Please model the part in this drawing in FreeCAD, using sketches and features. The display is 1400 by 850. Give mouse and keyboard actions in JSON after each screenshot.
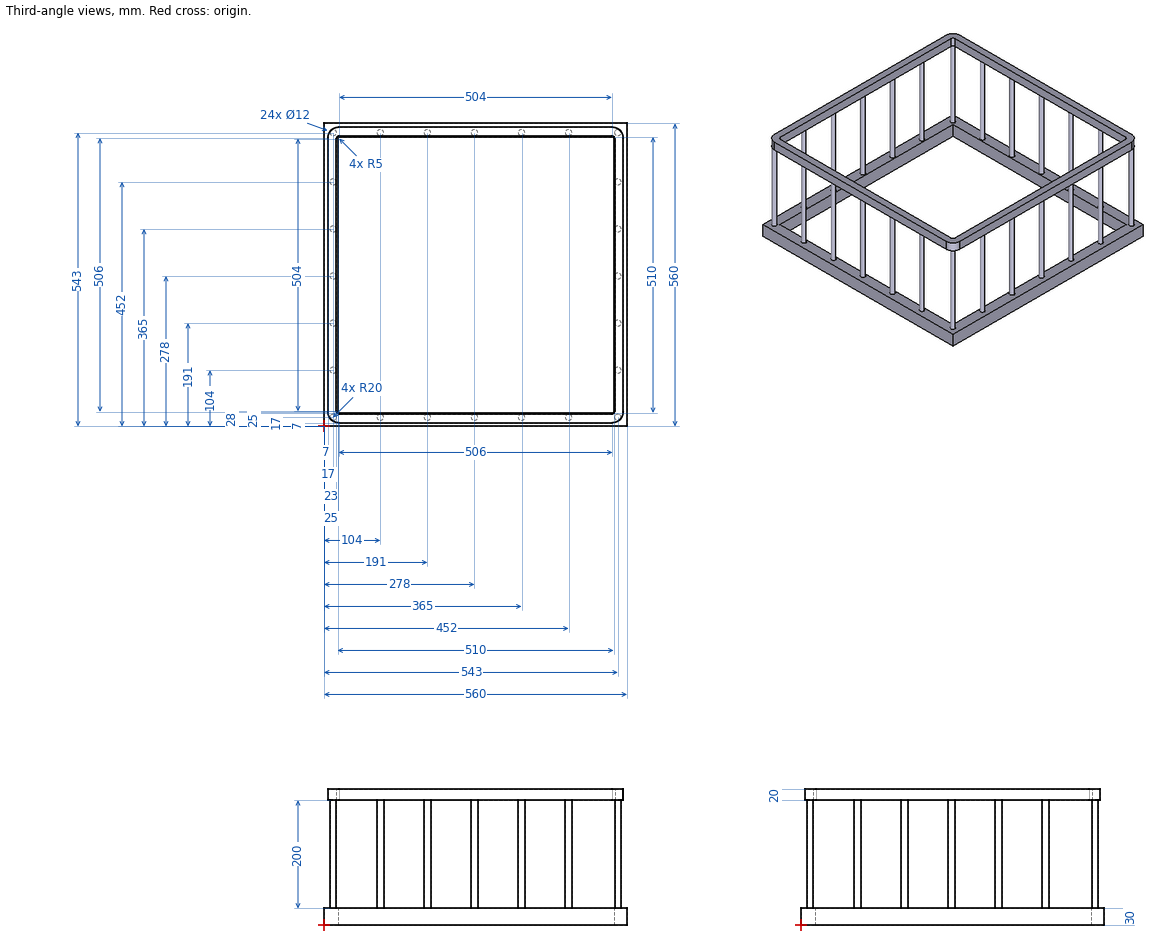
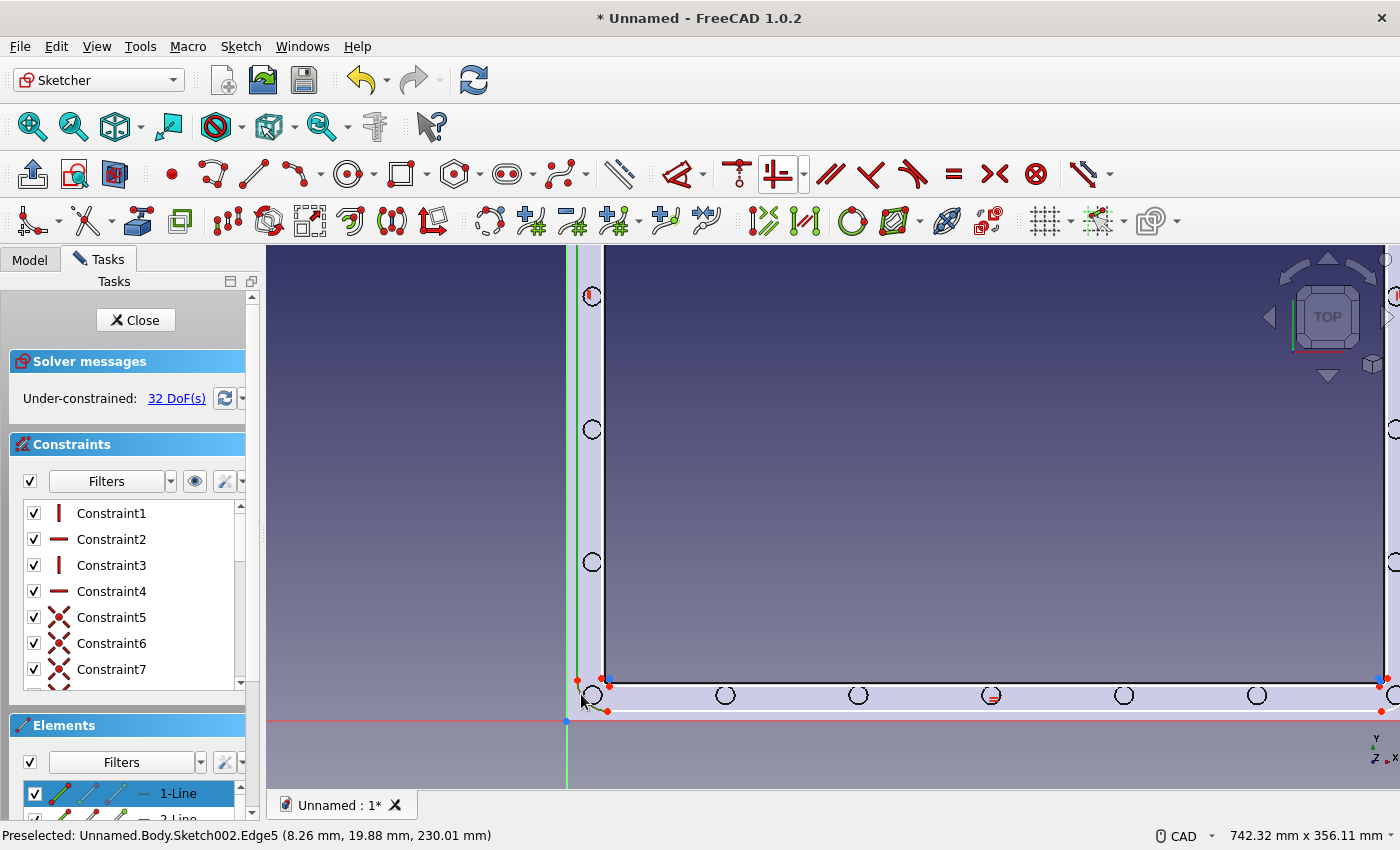
{"action": "left_click", "coordinate": [913, 174]}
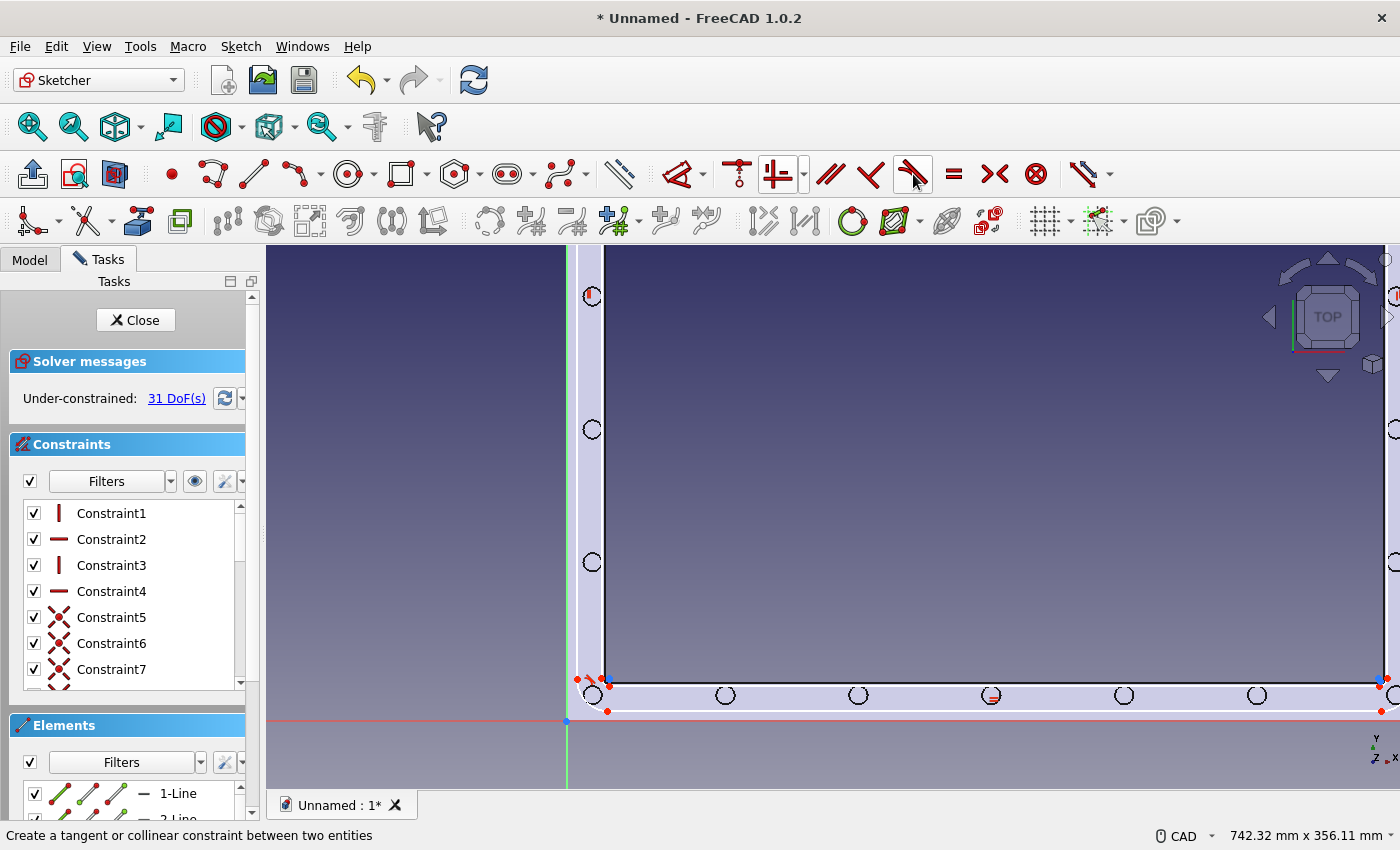
{"action": "scroll", "coordinate": [577, 448], "scroll_direction": "up", "scroll_amount": 2}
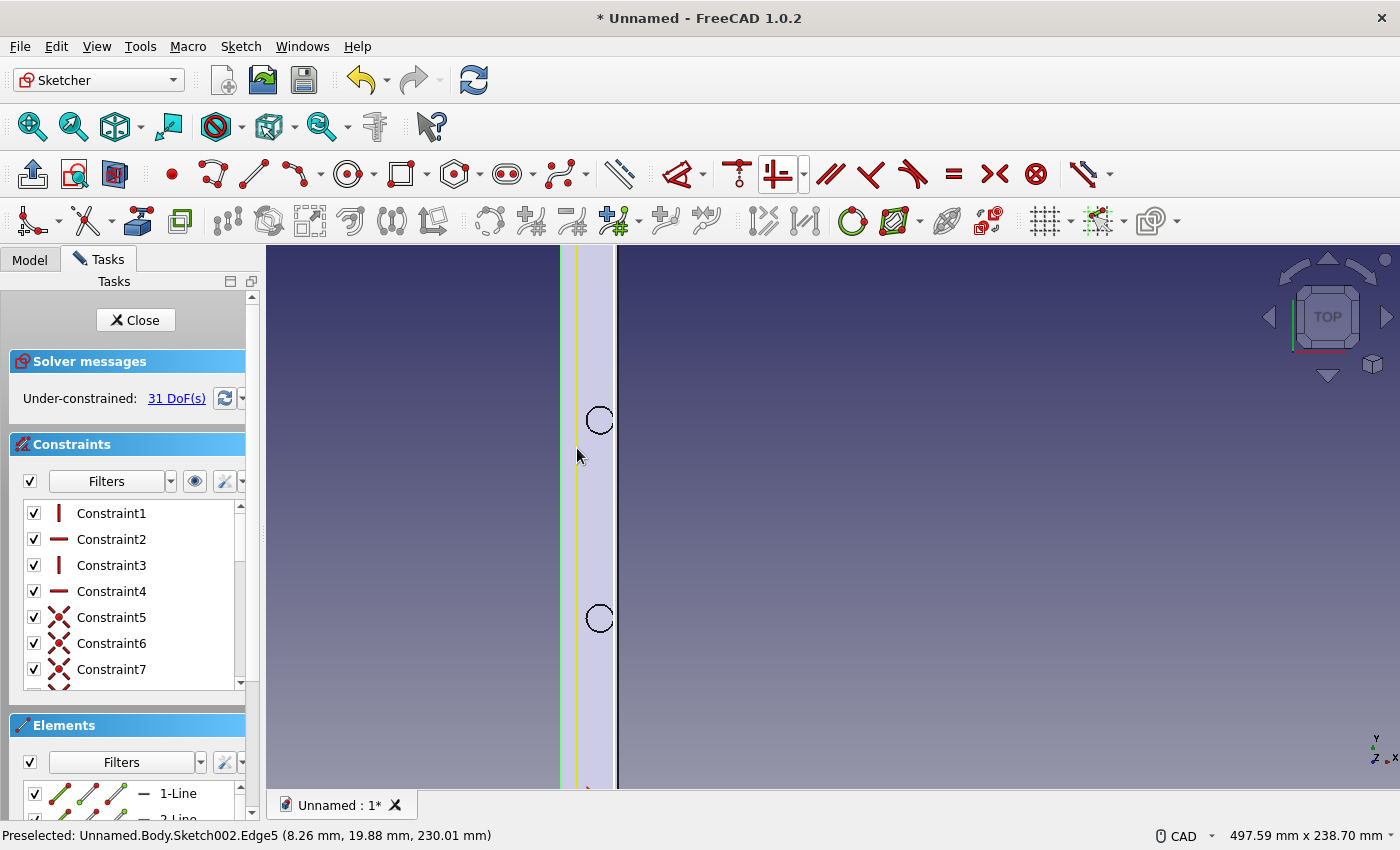
{"action": "left_click", "coordinate": [577, 448]}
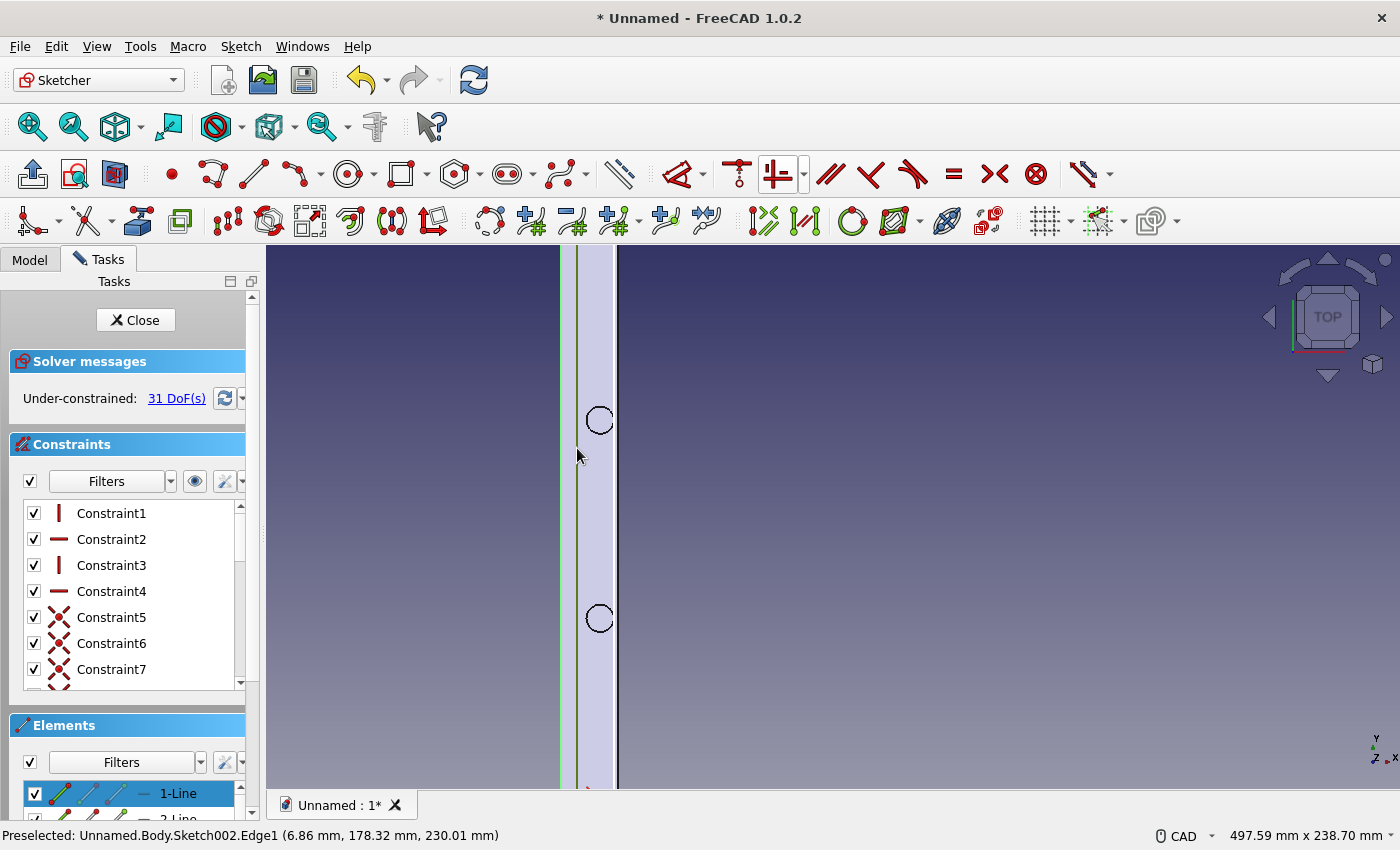
{"action": "scroll", "coordinate": [580, 643], "scroll_direction": "down", "scroll_amount": 6}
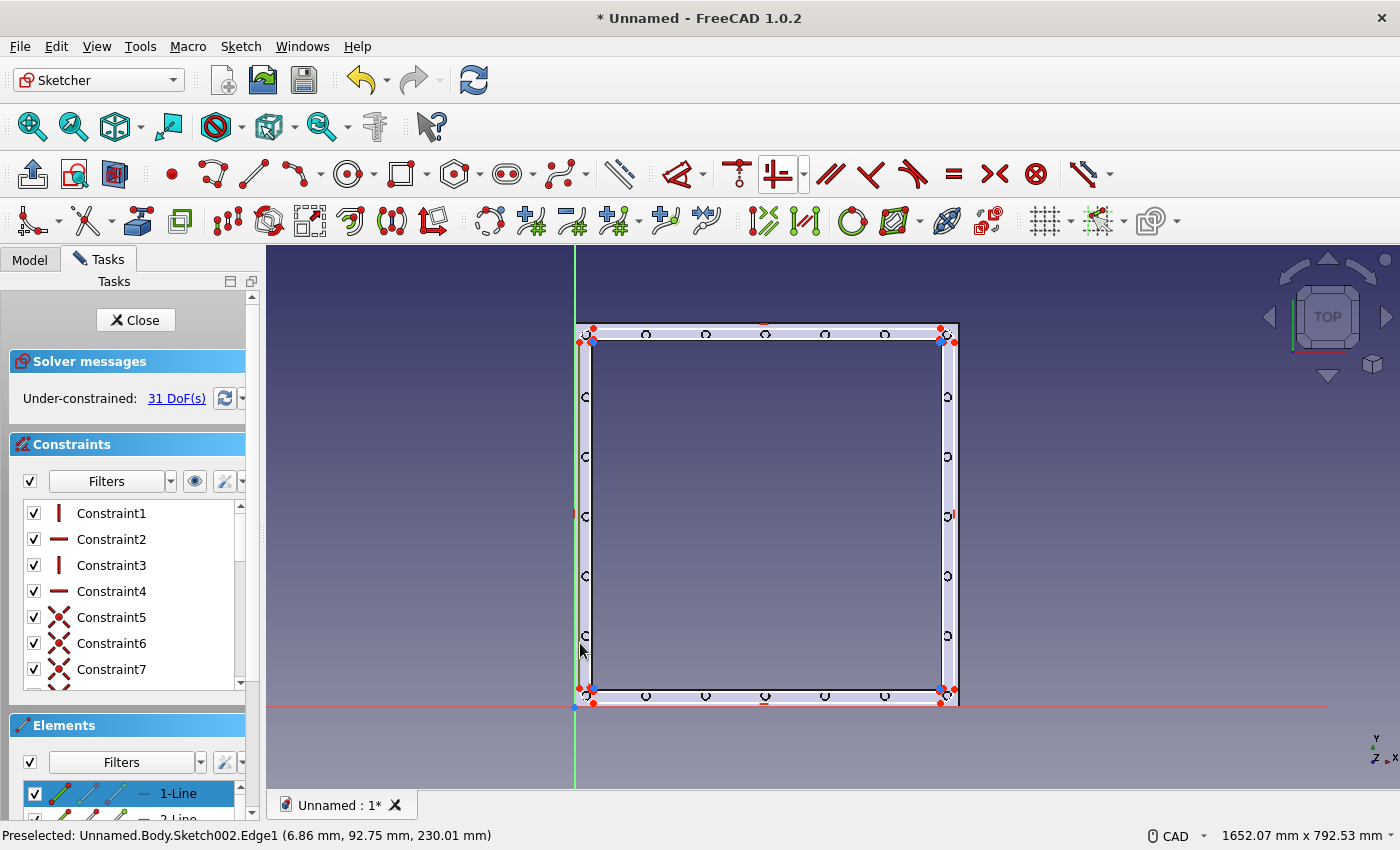
{"action": "scroll", "coordinate": [587, 330], "scroll_direction": "up", "scroll_amount": 4}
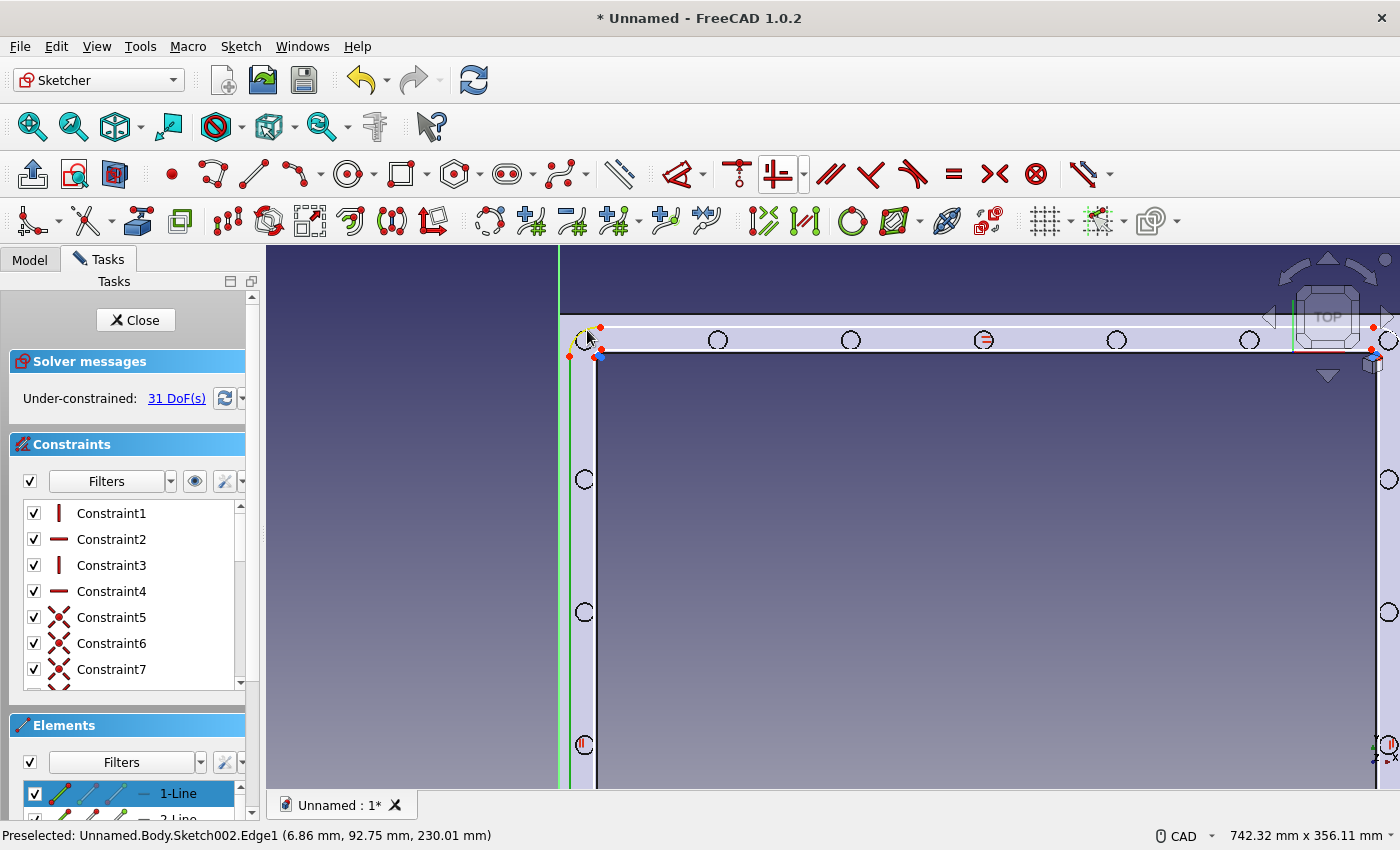
{"action": "left_click", "coordinate": [587, 330]}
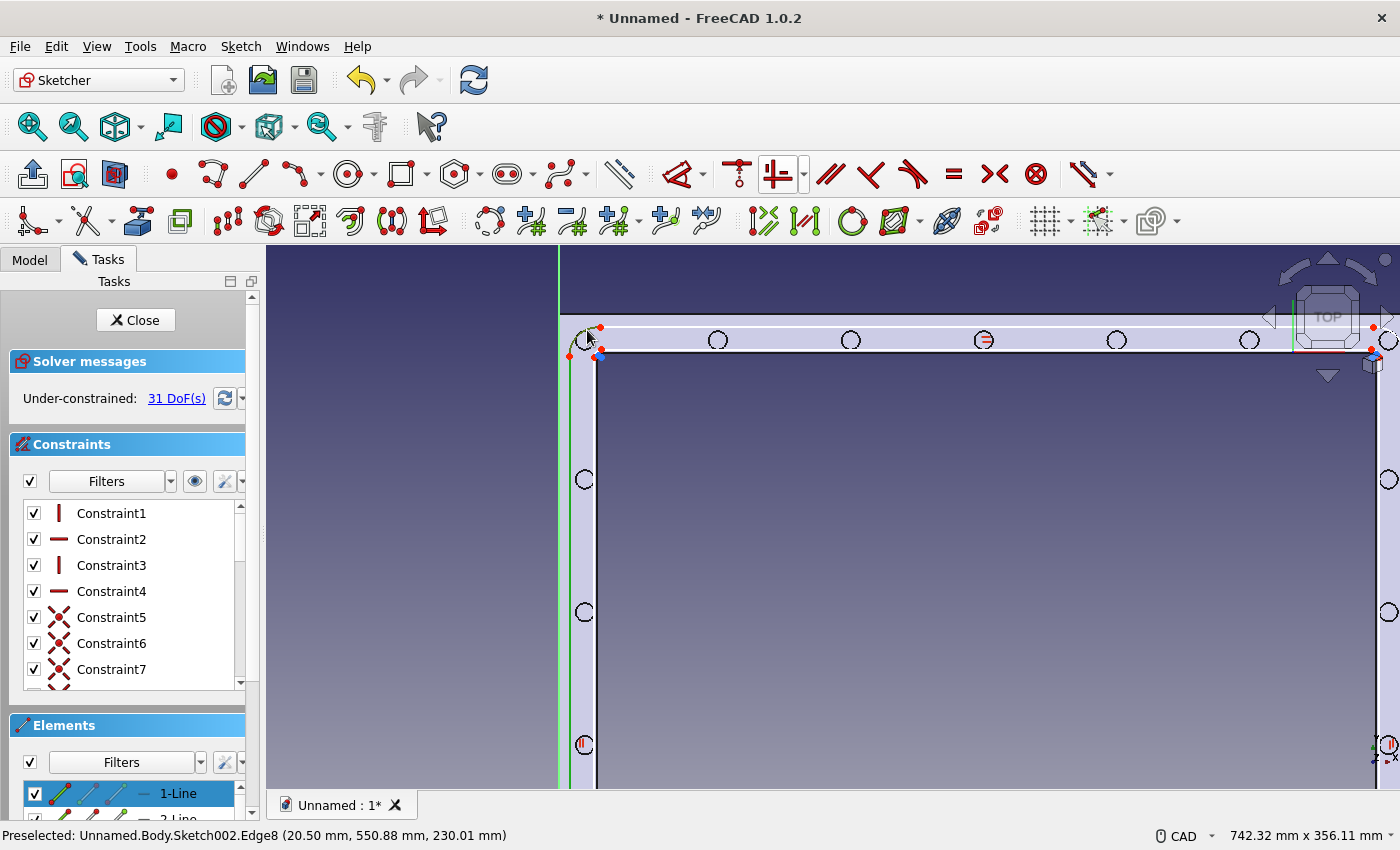
{"action": "left_click", "coordinate": [913, 174]}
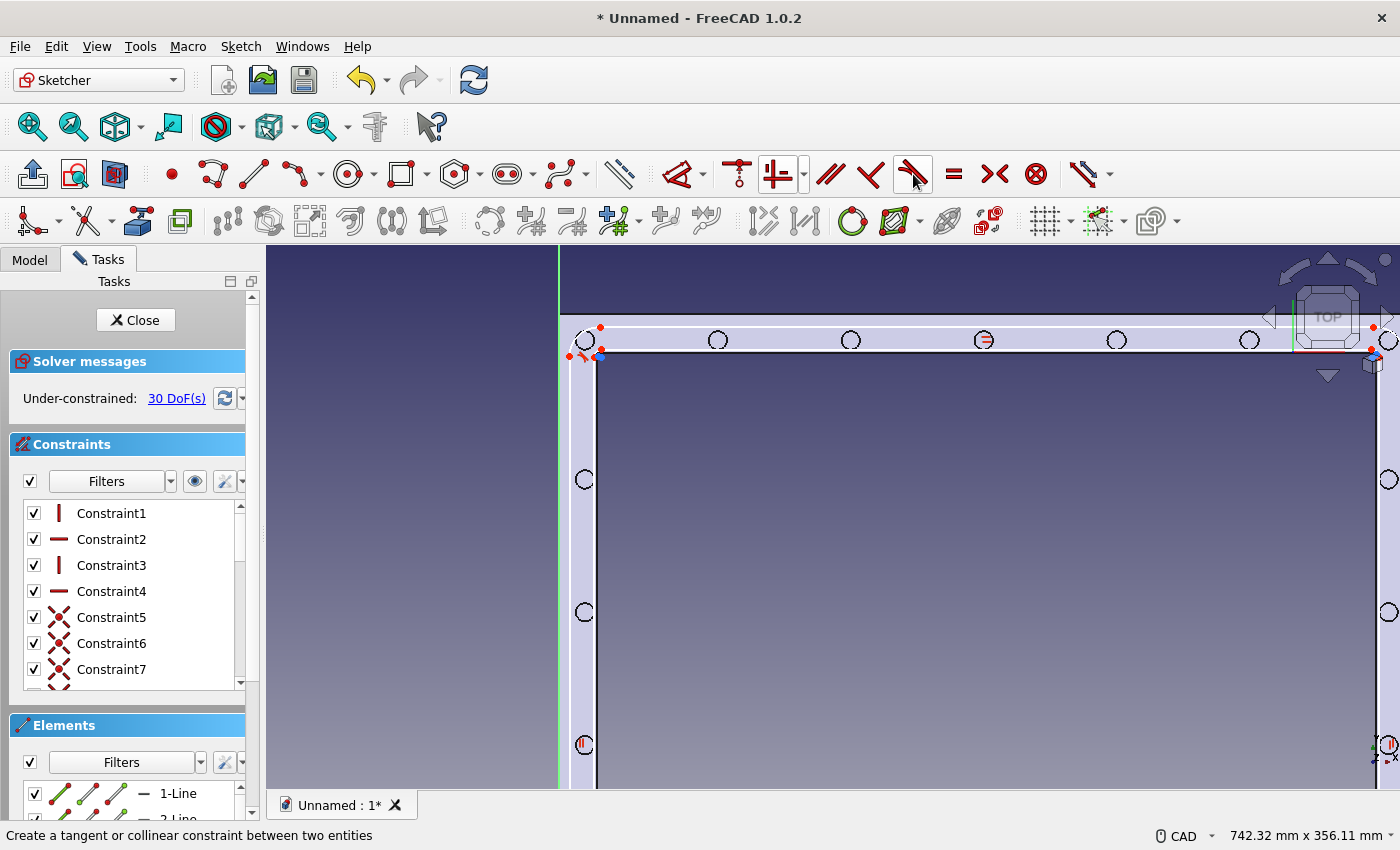
{"action": "scroll", "coordinate": [587, 329], "scroll_direction": "down", "scroll_amount": 4}